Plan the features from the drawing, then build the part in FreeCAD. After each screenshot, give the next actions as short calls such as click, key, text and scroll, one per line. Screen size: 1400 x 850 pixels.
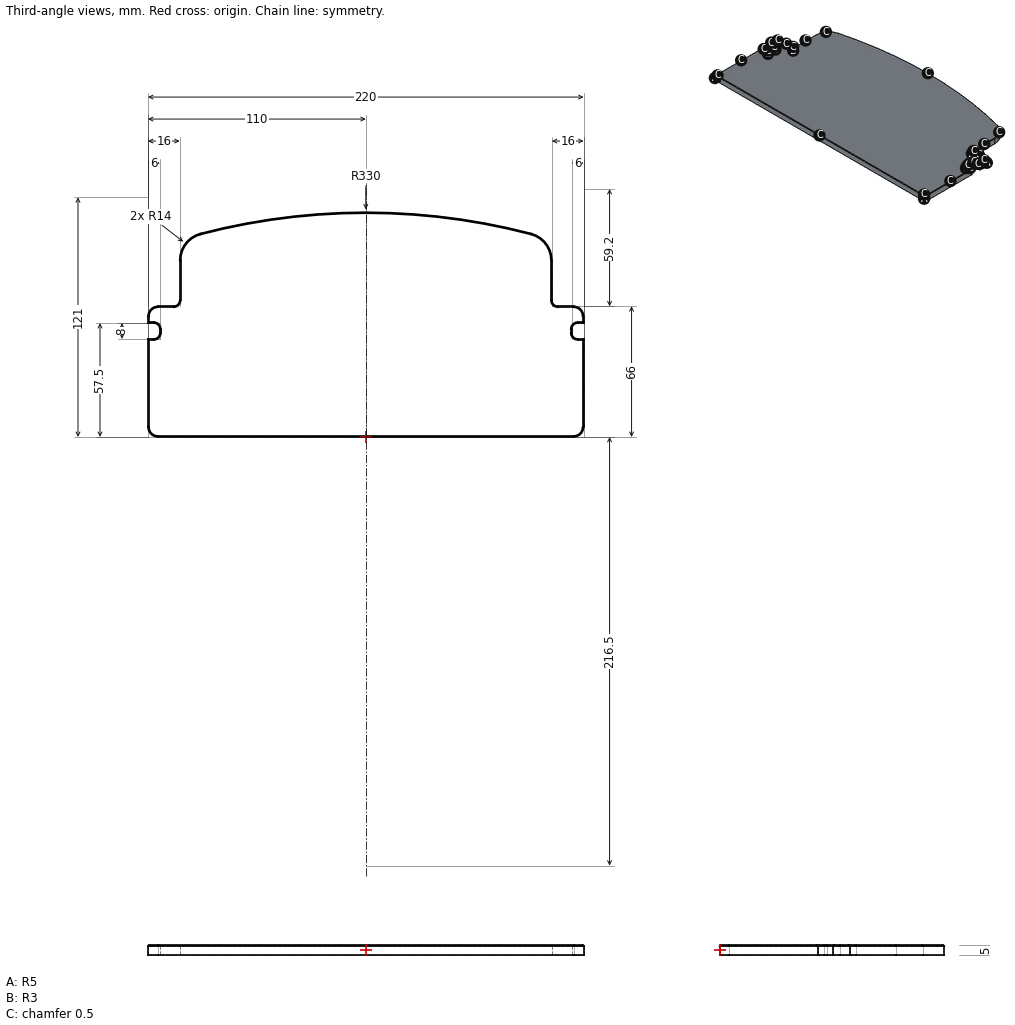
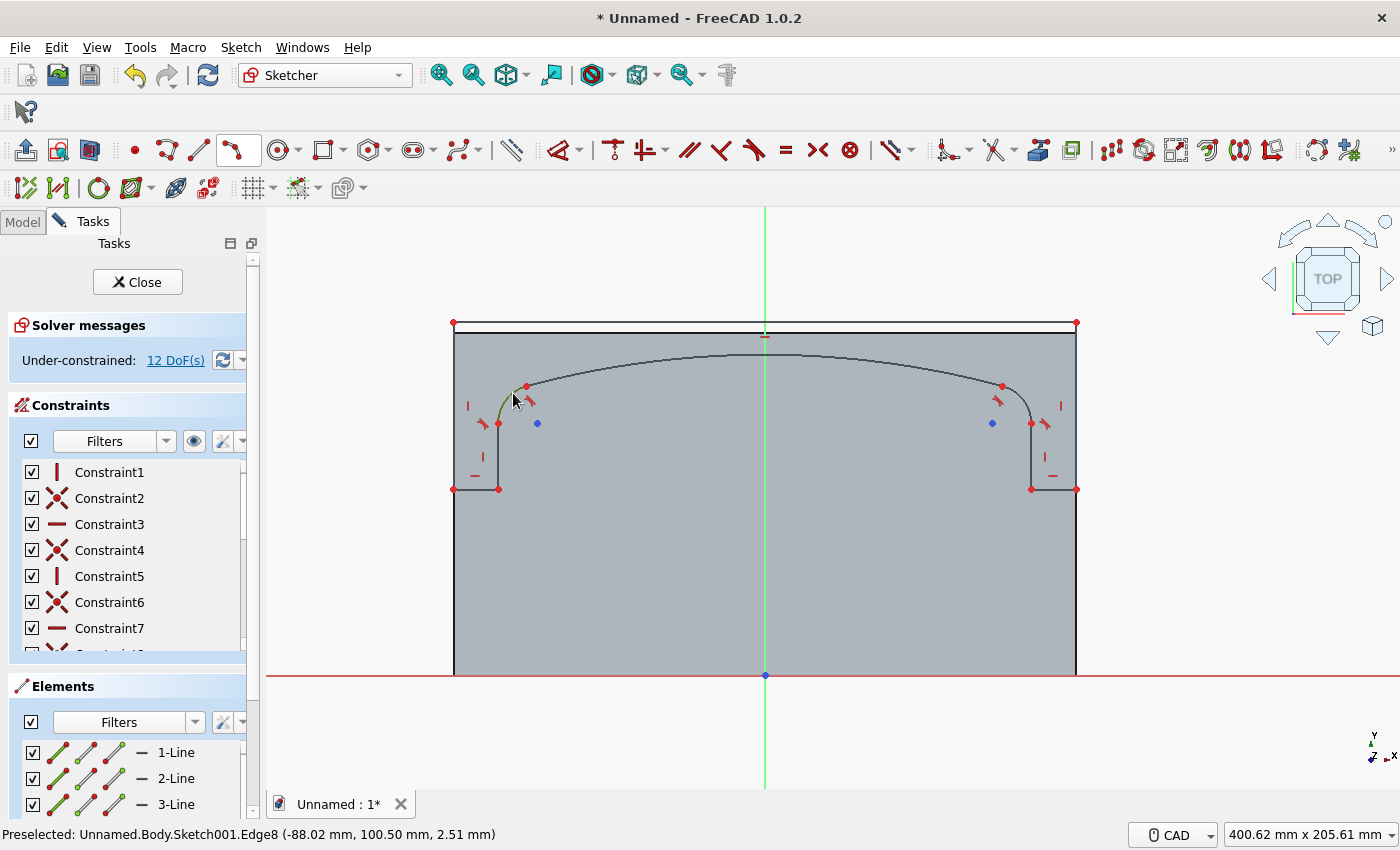
click(1028, 409)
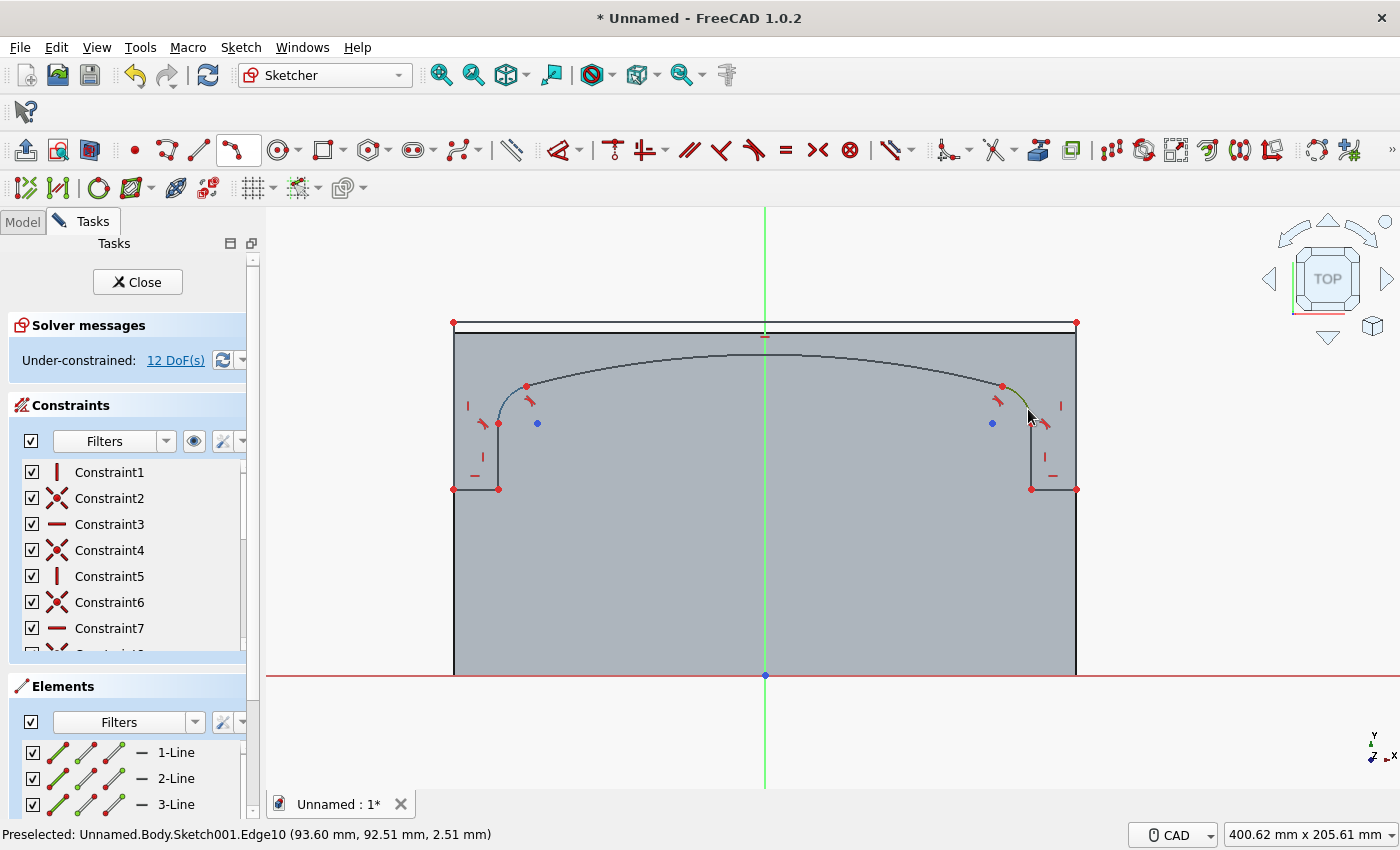
key(e)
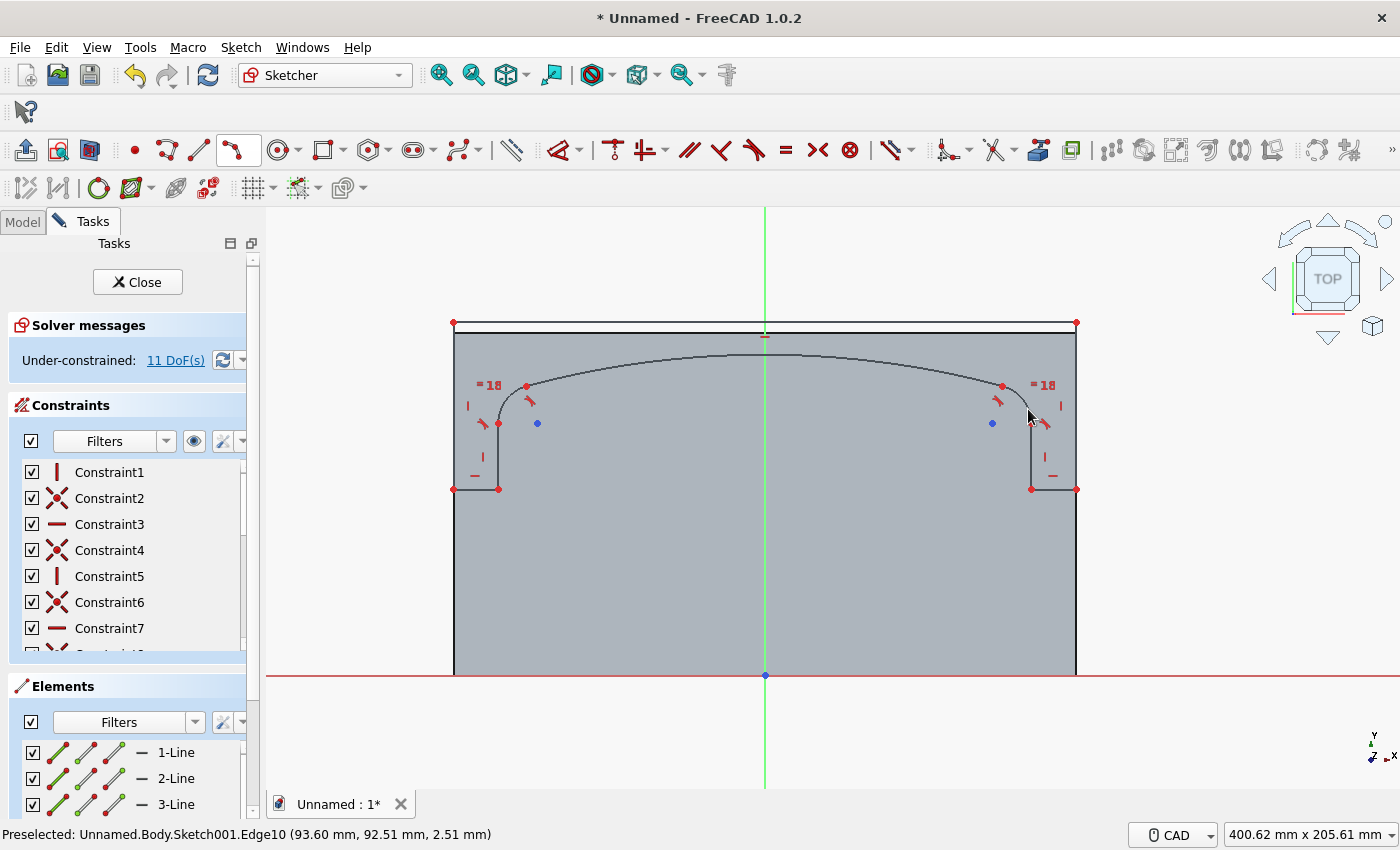
scroll(764, 325, down, 5)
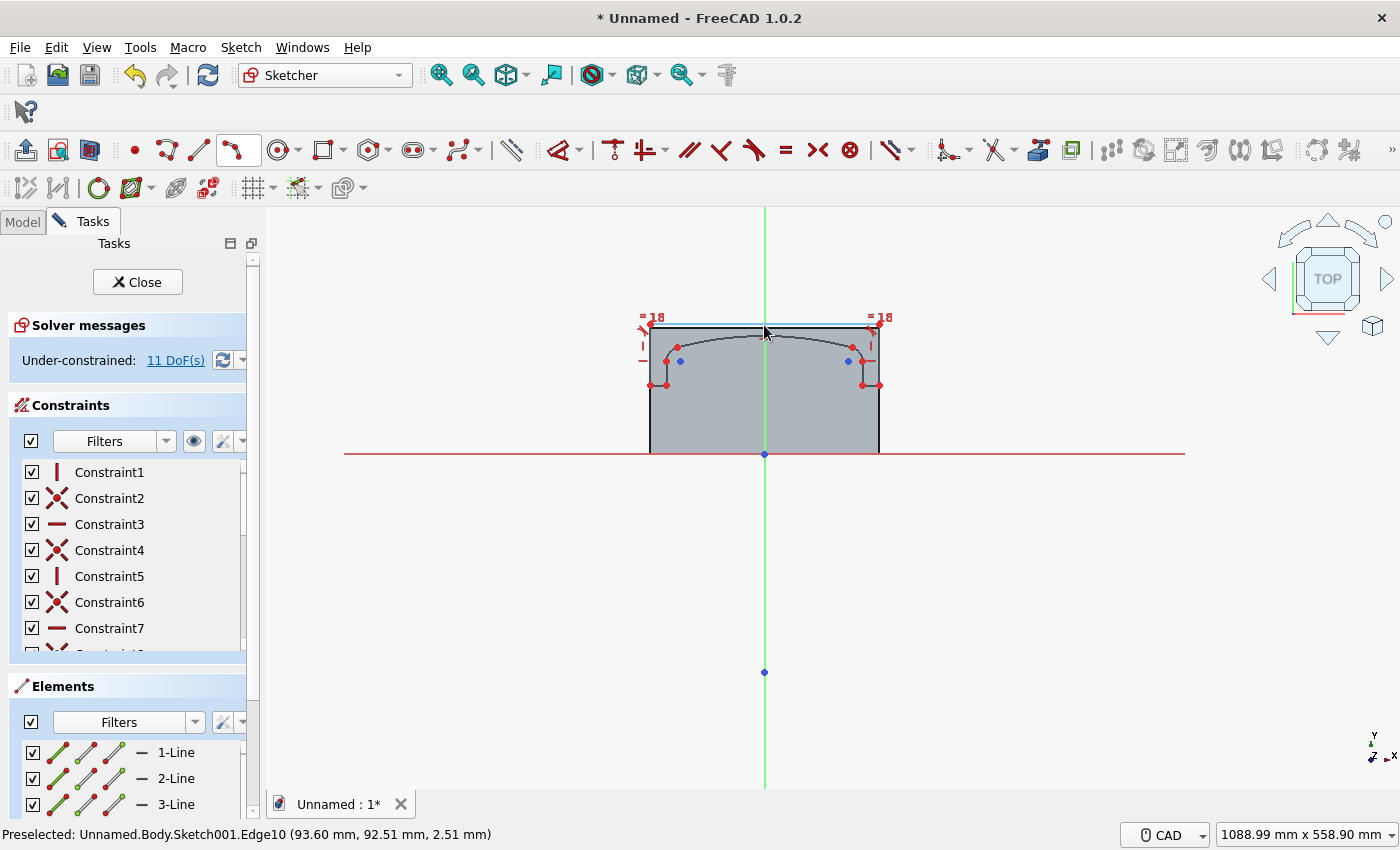
click(764, 673)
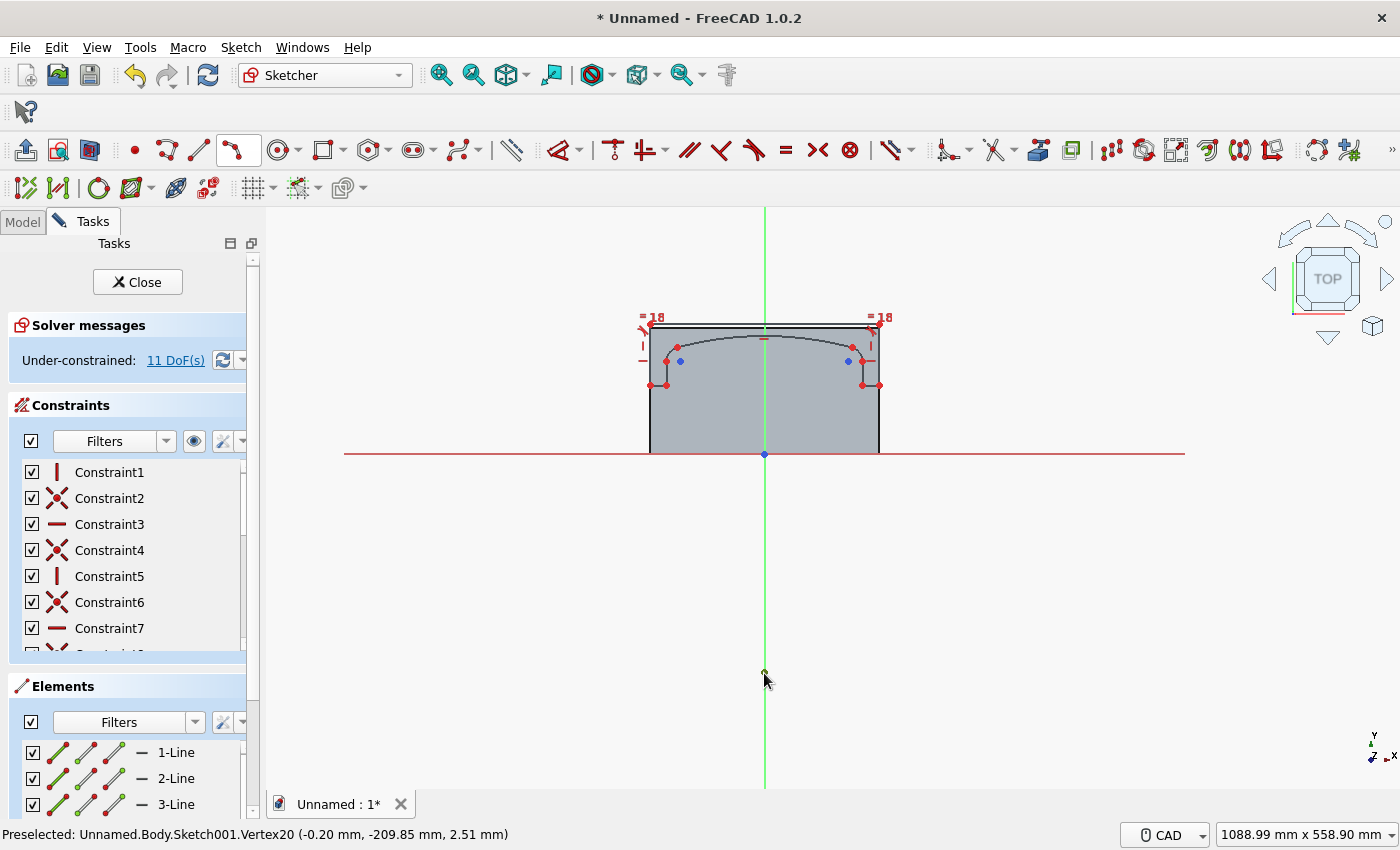
click(765, 723)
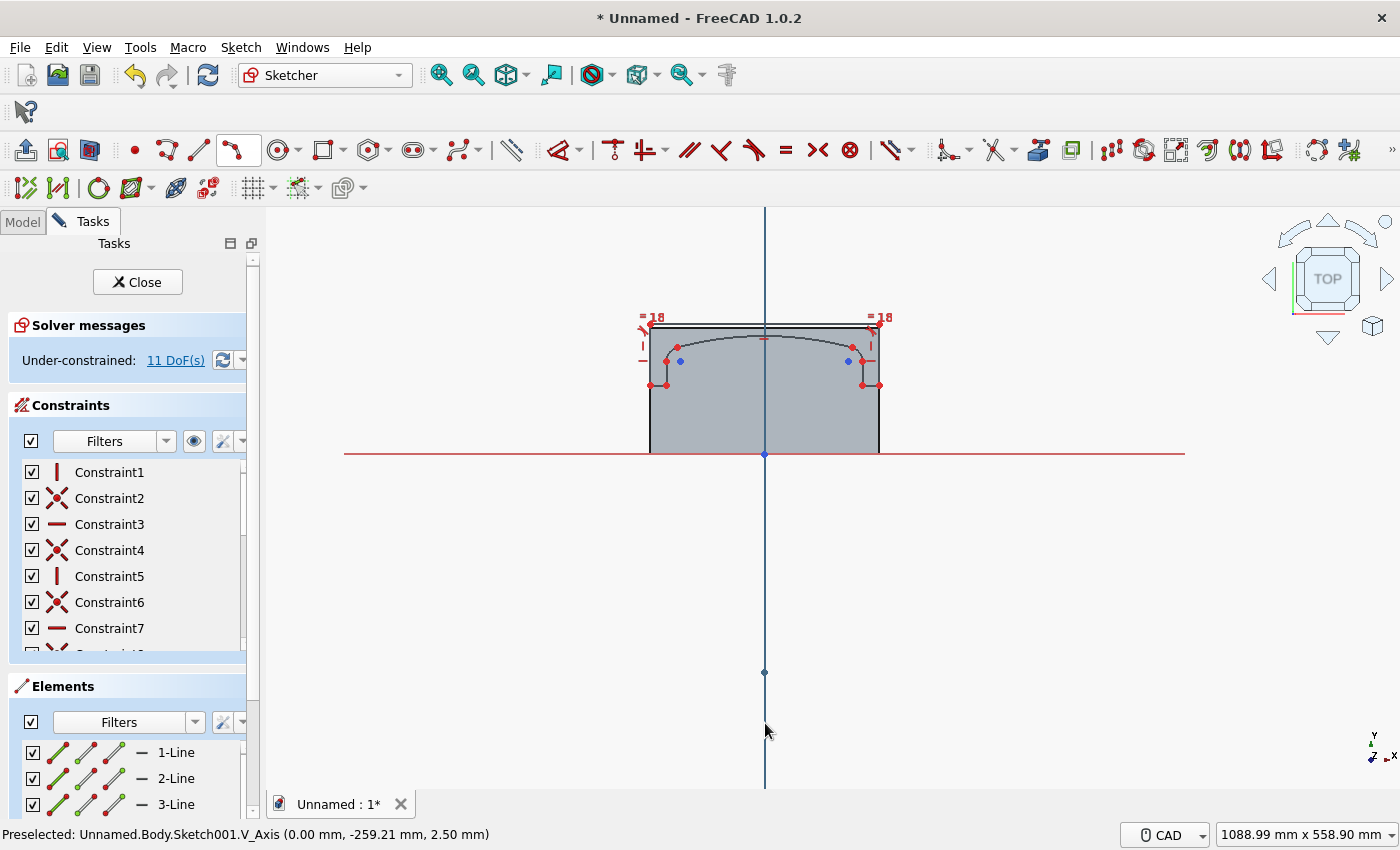
click(614, 150)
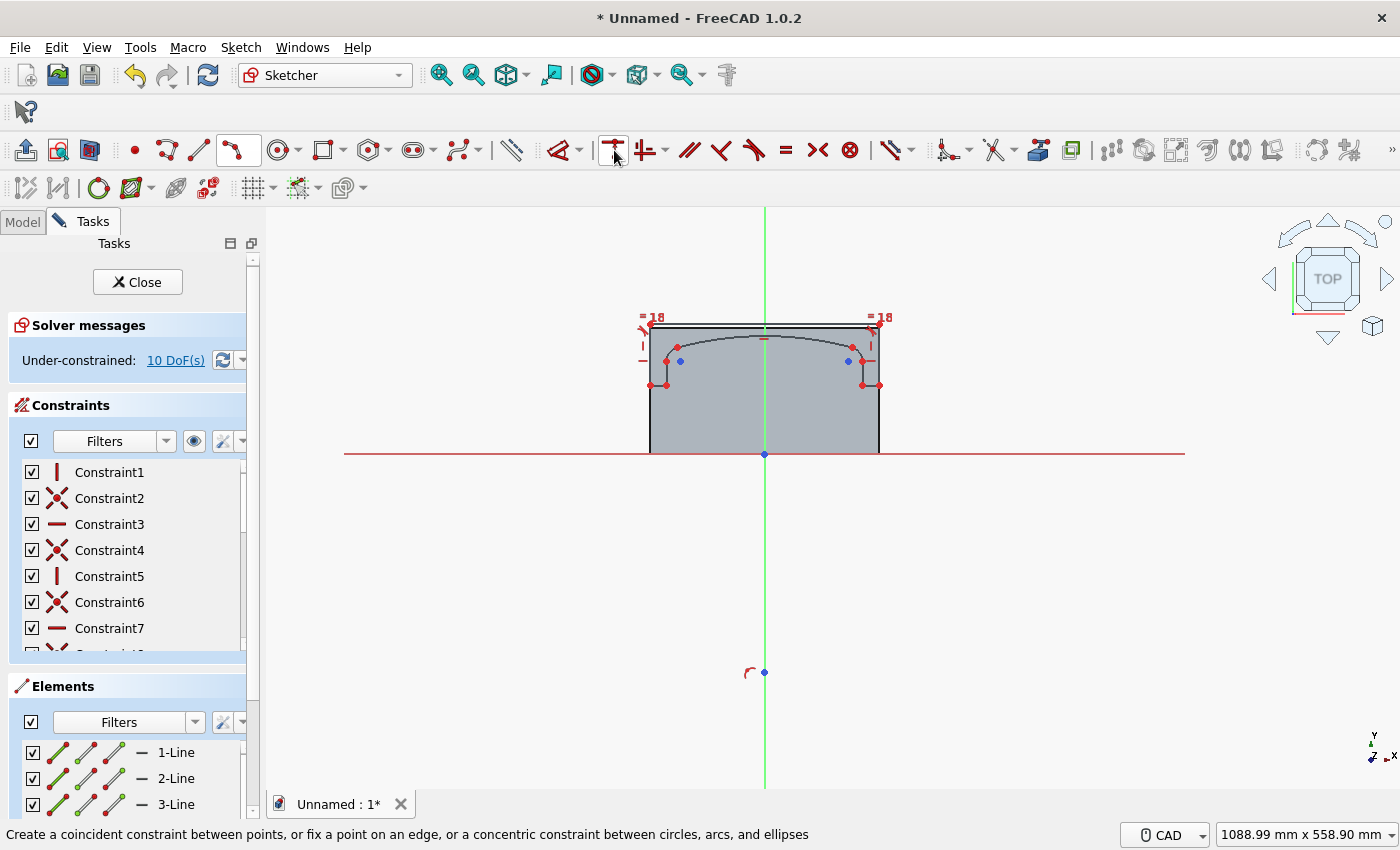
click(879, 386)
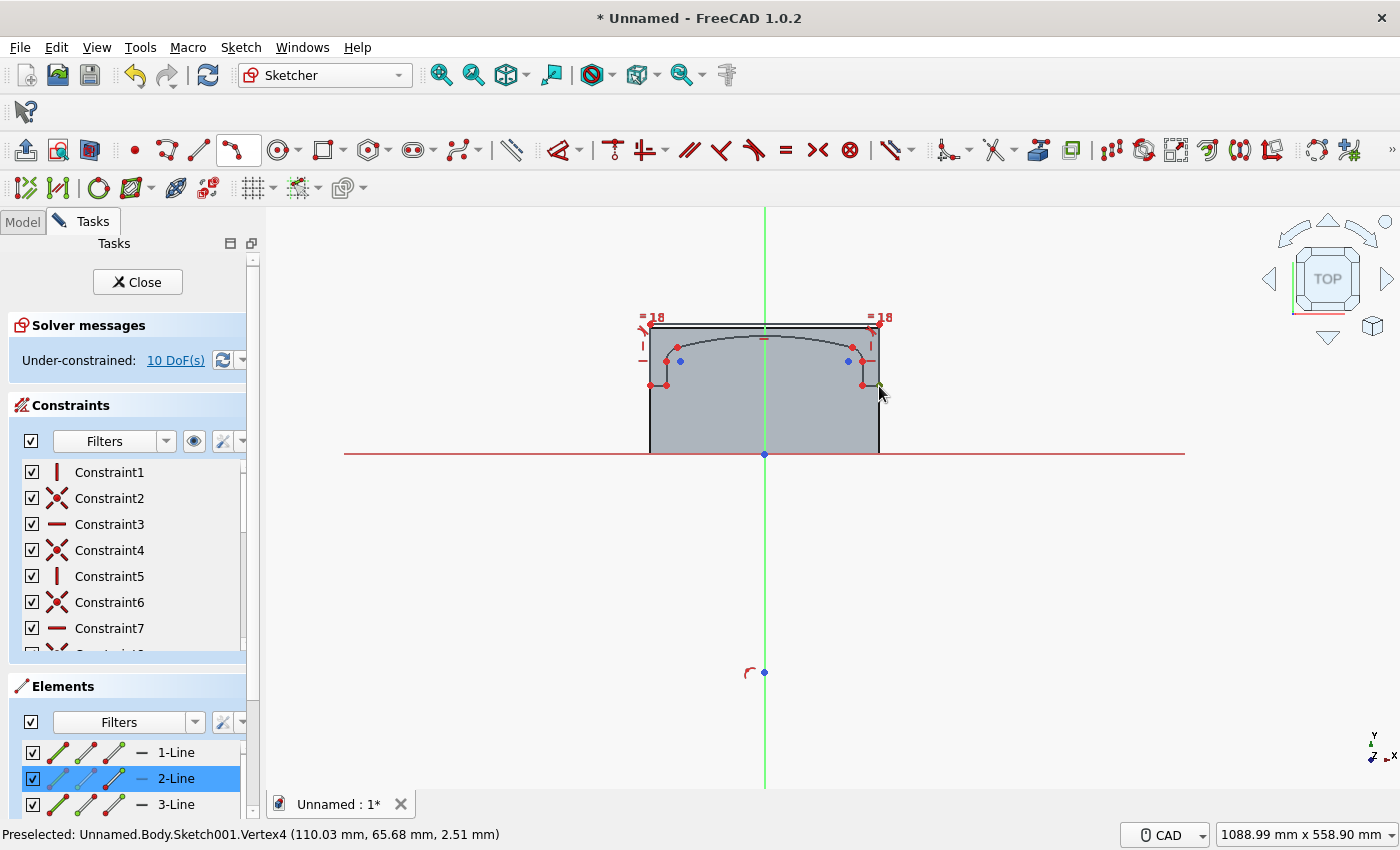
click(650, 386)